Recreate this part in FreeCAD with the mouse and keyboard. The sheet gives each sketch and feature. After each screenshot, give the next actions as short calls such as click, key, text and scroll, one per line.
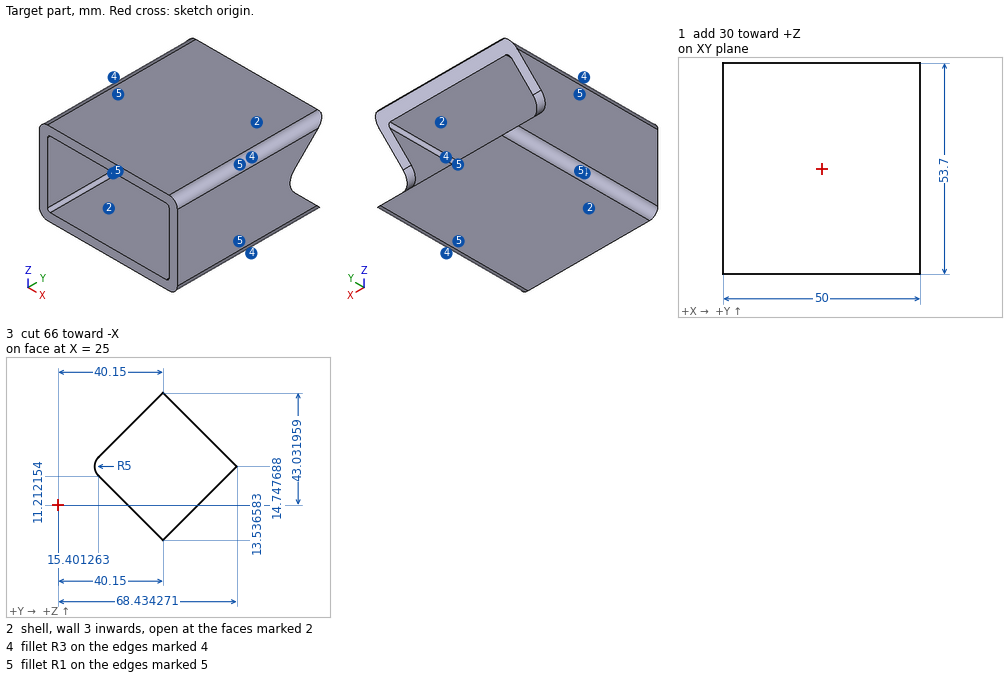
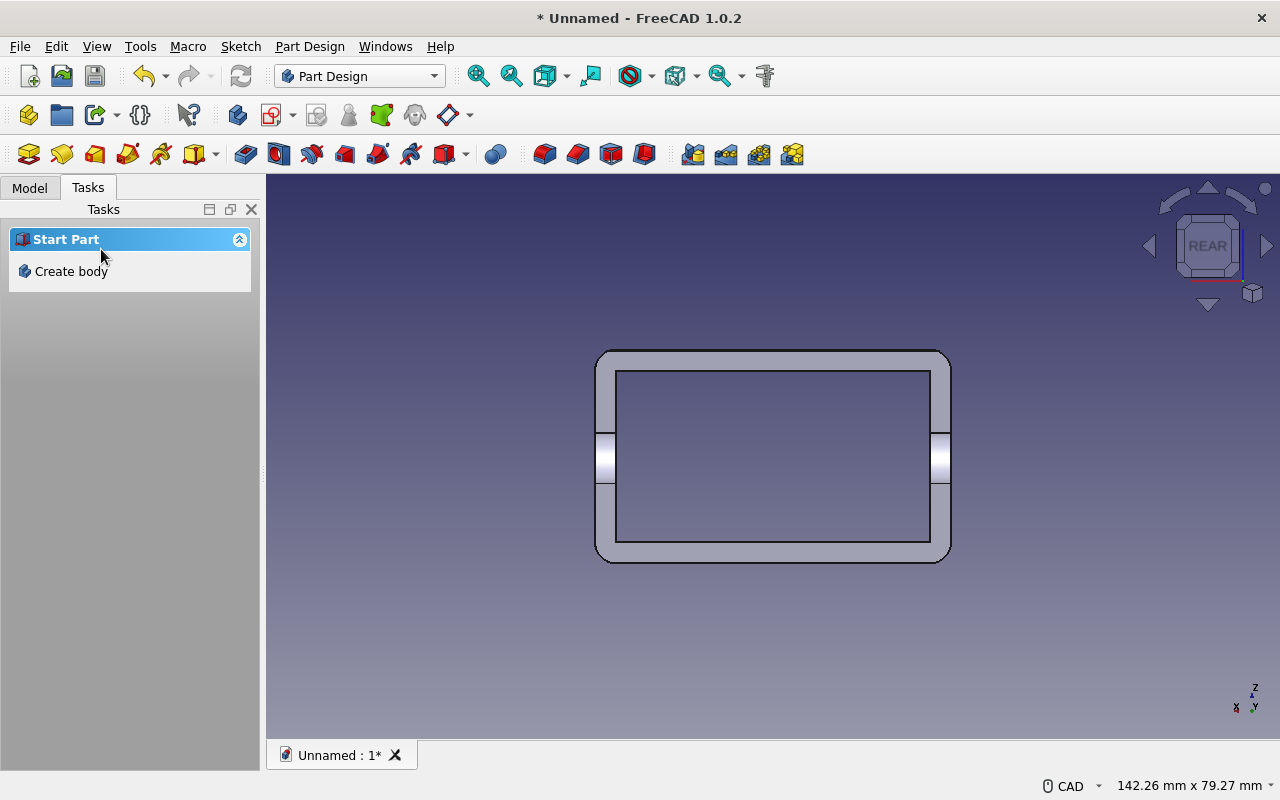
key(v)
key(f)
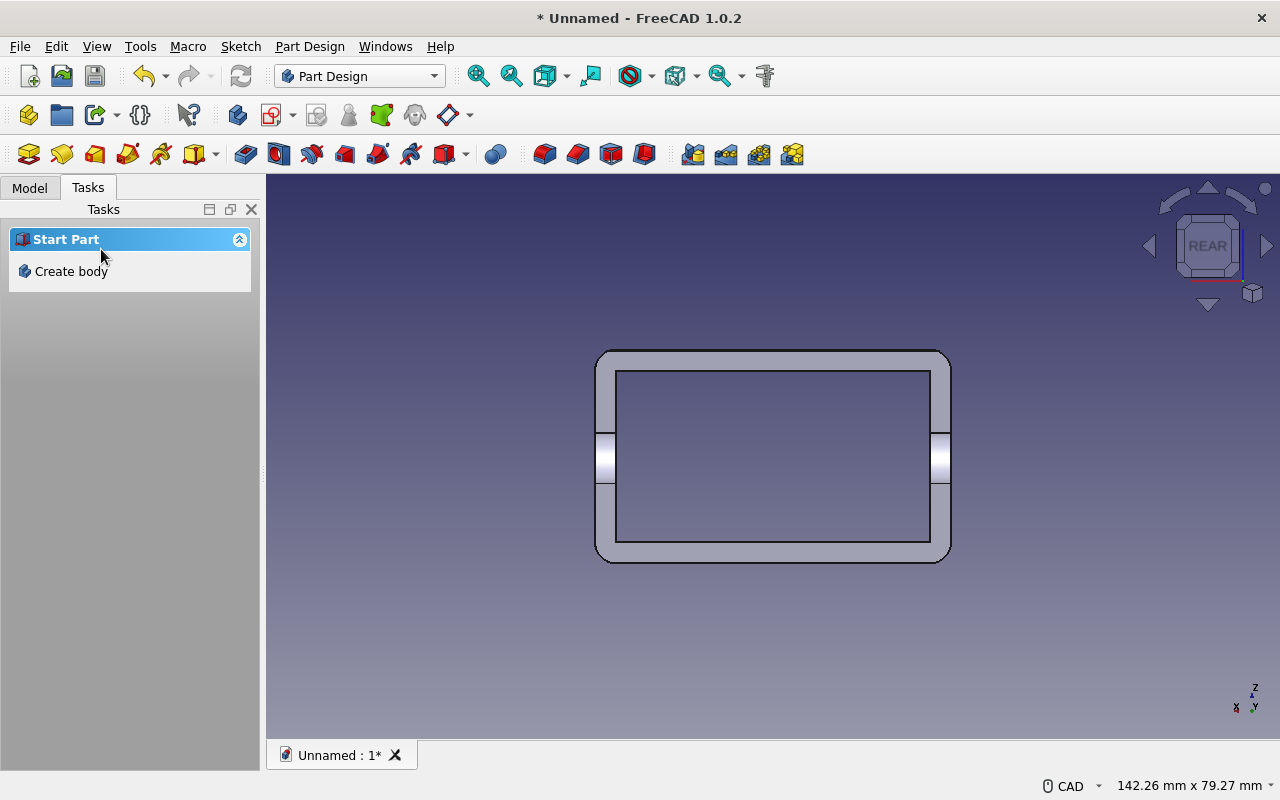
key(6)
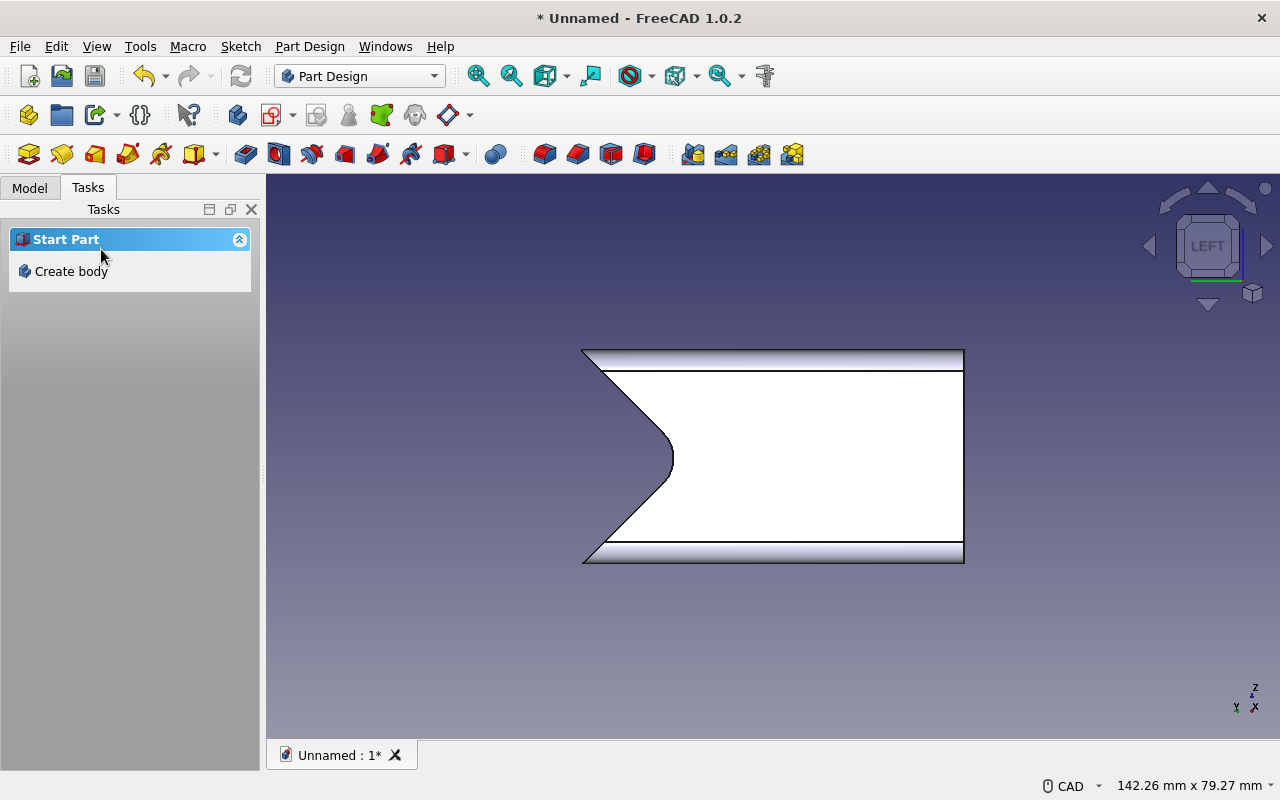
key(v)
key(f)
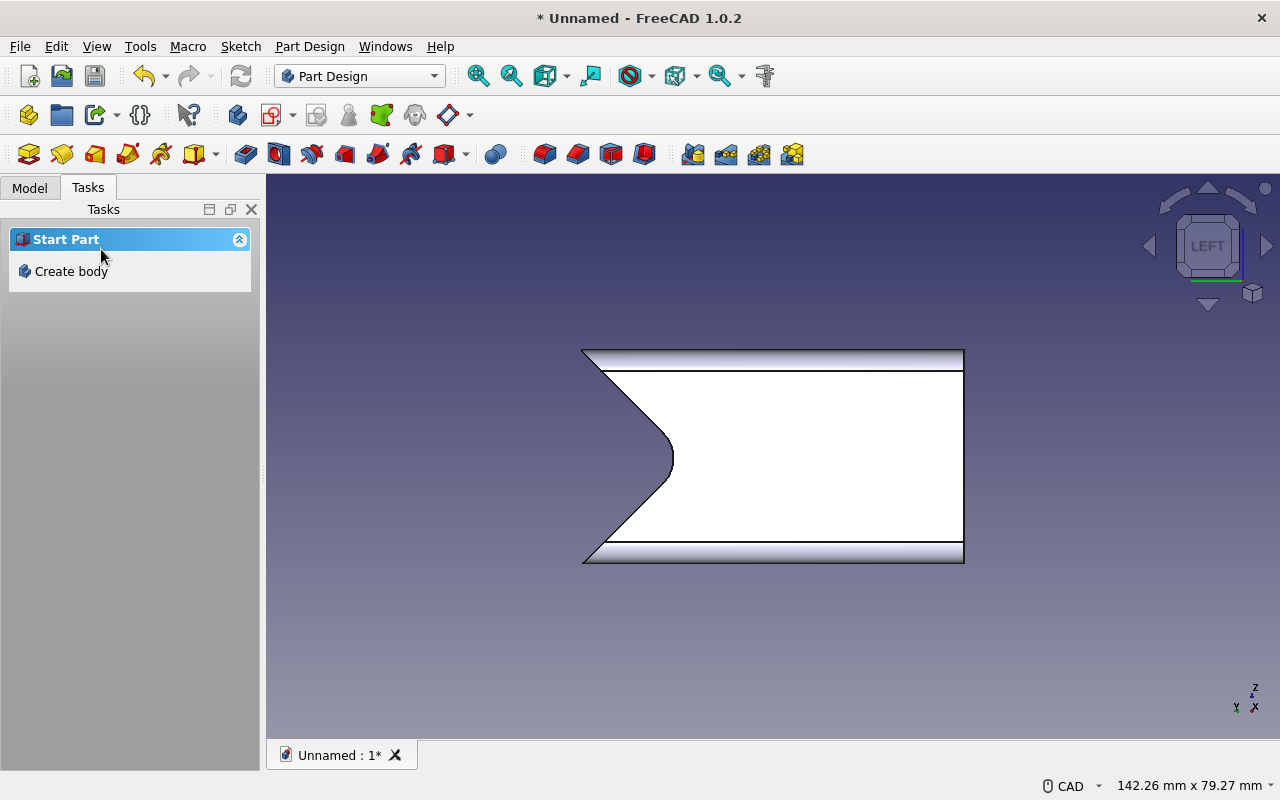
key(v)
key(3)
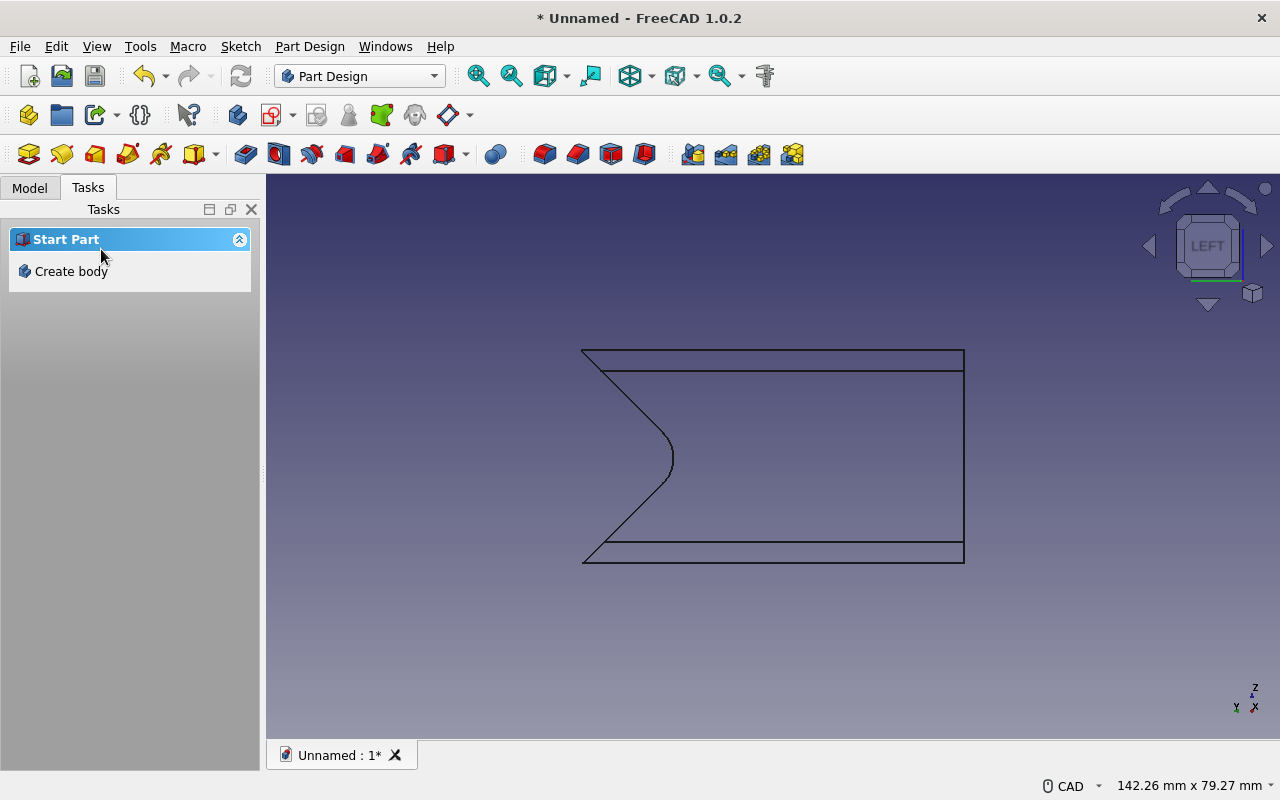
key(0)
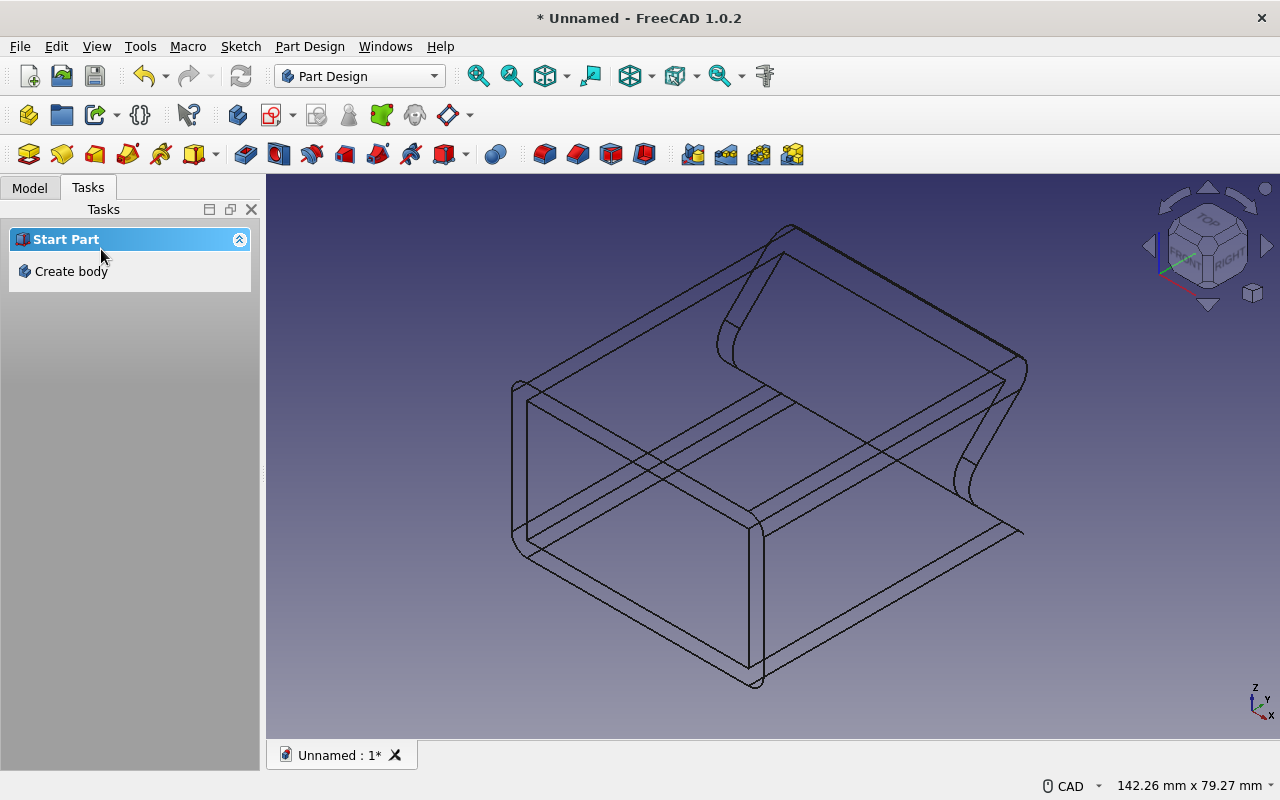
click(876, 594)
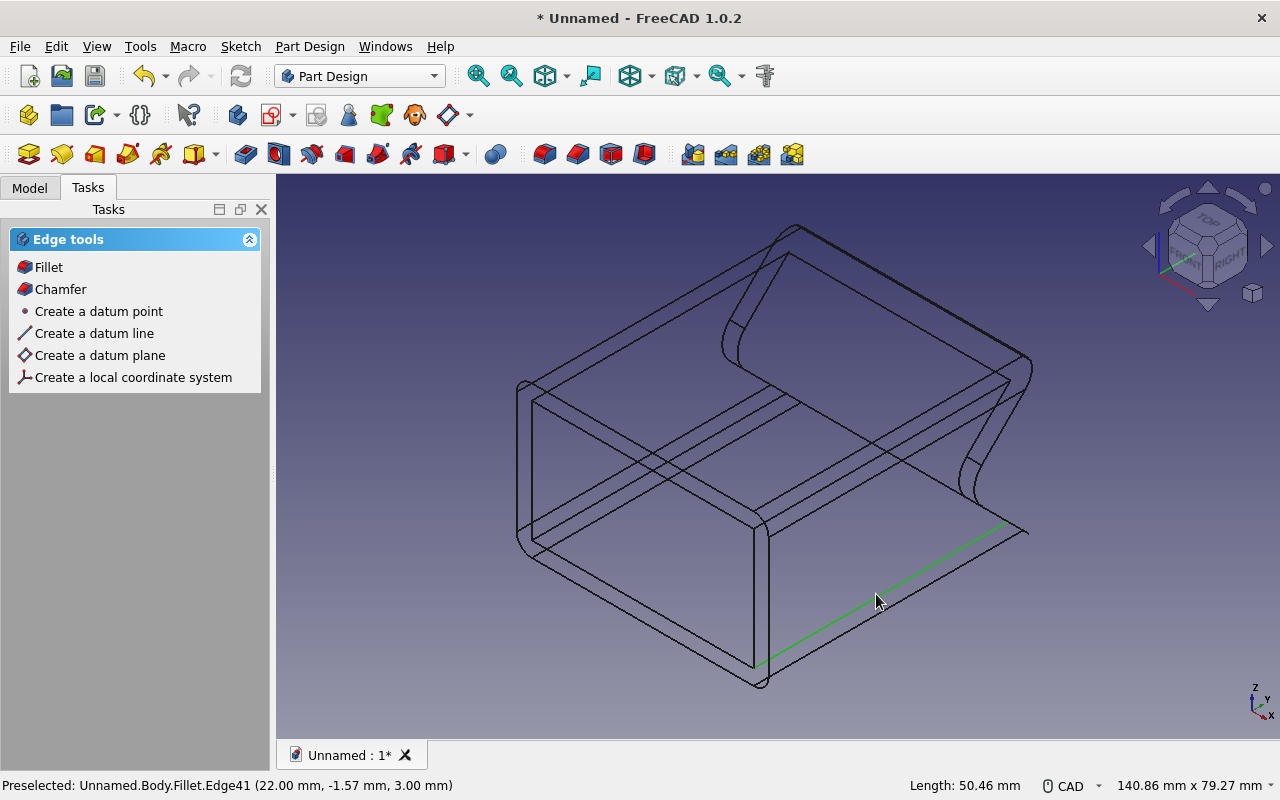
click(882, 454, ctrl)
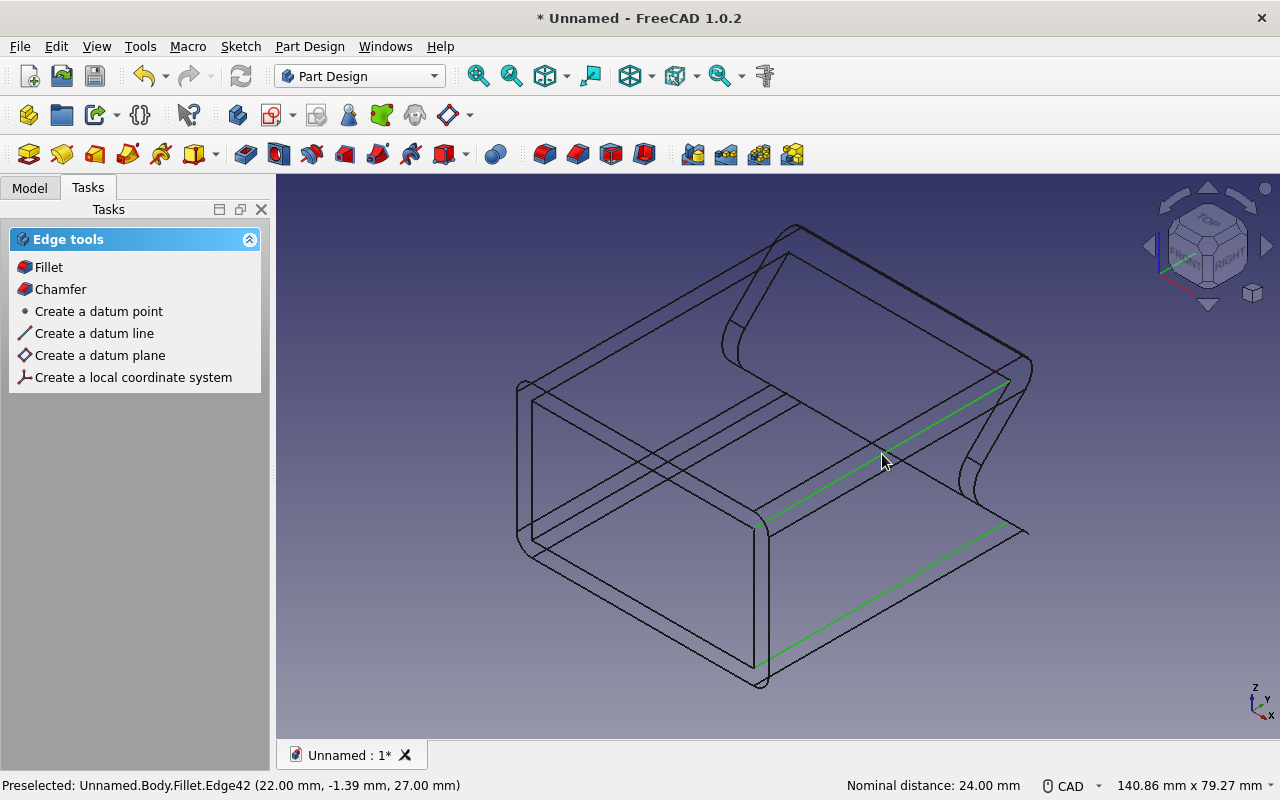
click(684, 451, ctrl)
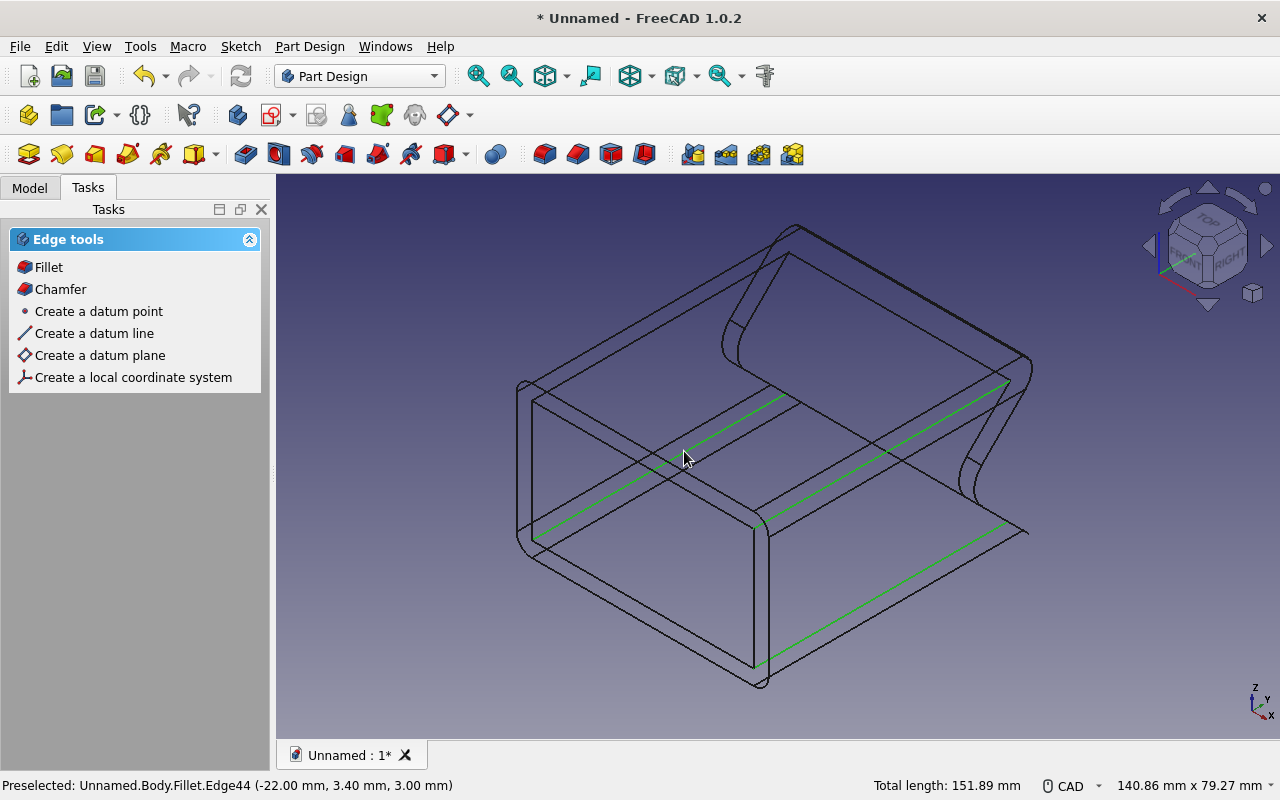
click(660, 326, ctrl)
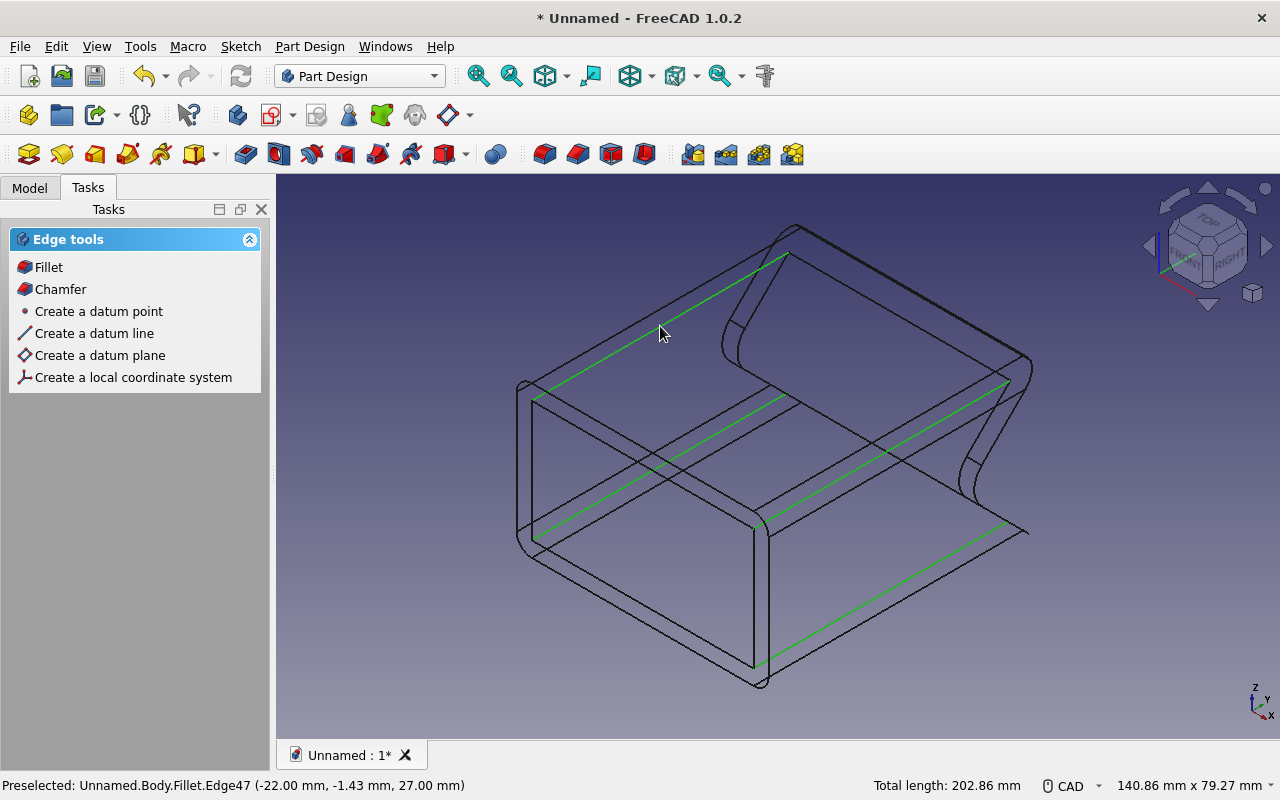
key(v)
key(1)